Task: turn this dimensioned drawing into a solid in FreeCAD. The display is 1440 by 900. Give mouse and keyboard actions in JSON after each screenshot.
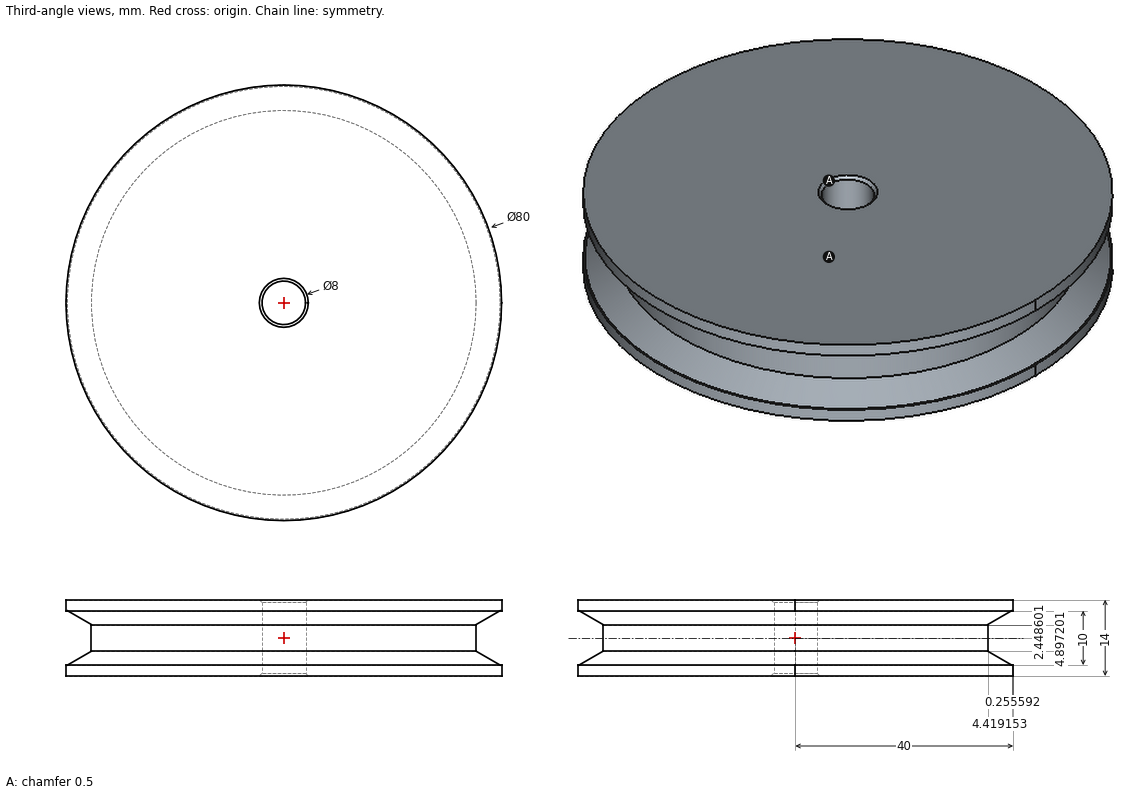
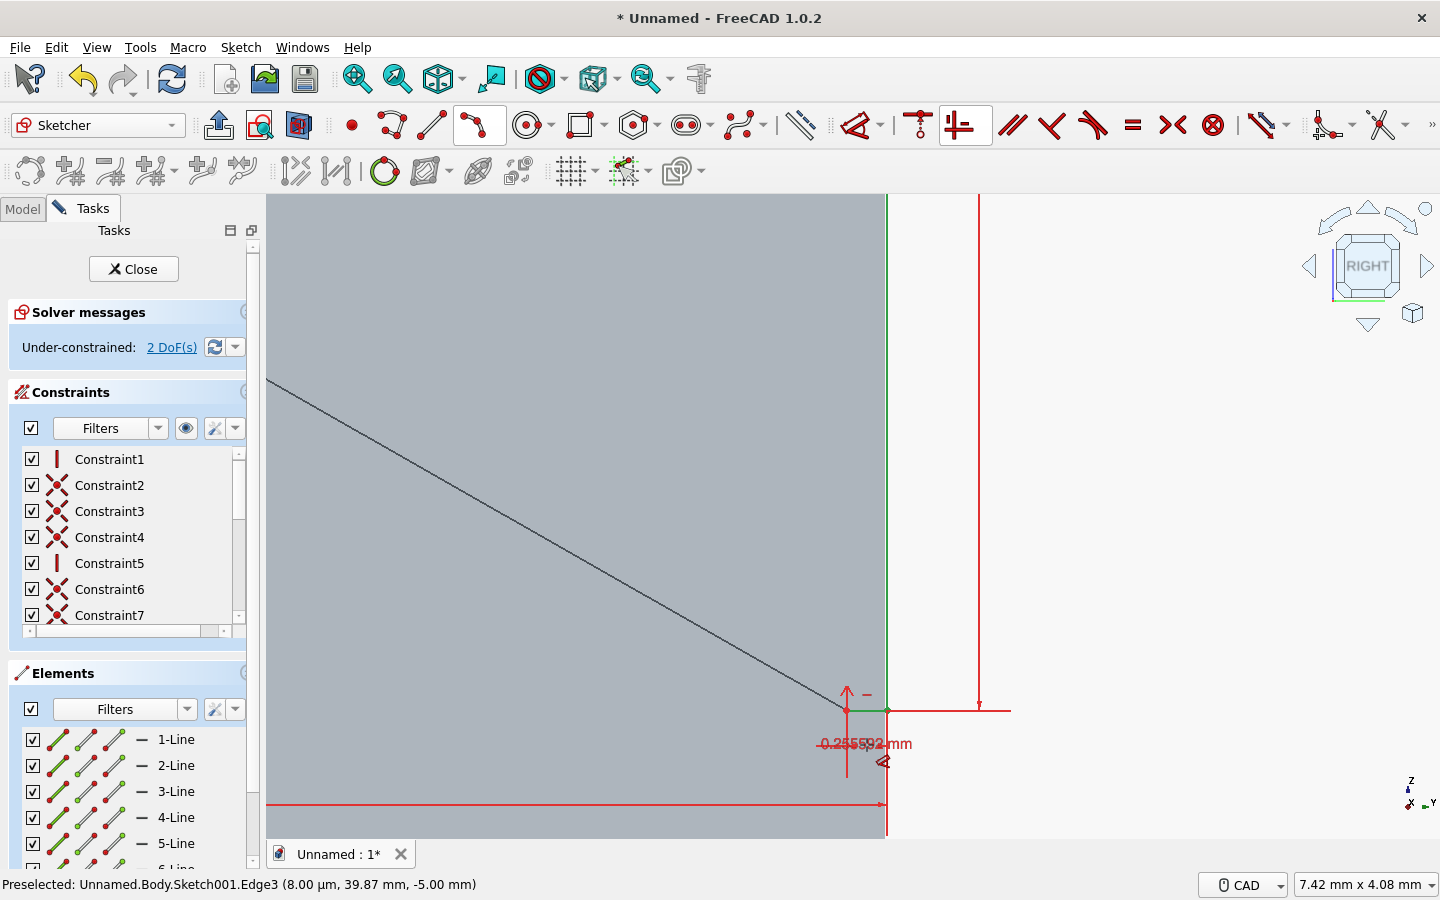
{"action": "scroll", "coordinate": [872, 712], "scroll_direction": "down", "scroll_amount": 7}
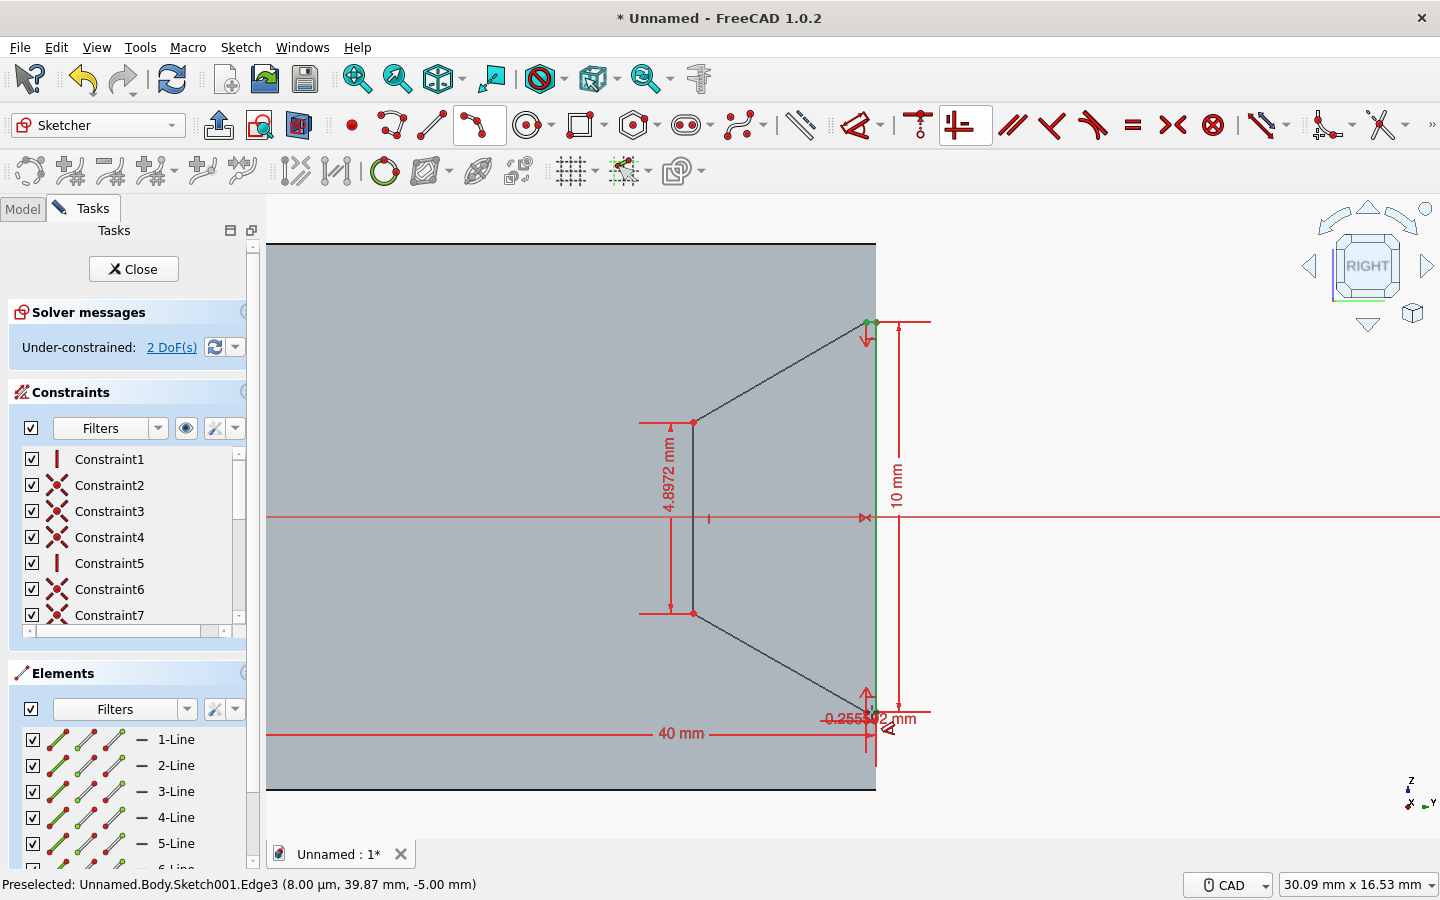
{"action": "left_click", "coordinate": [693, 423]}
{"action": "left_click", "coordinate": [727, 448]}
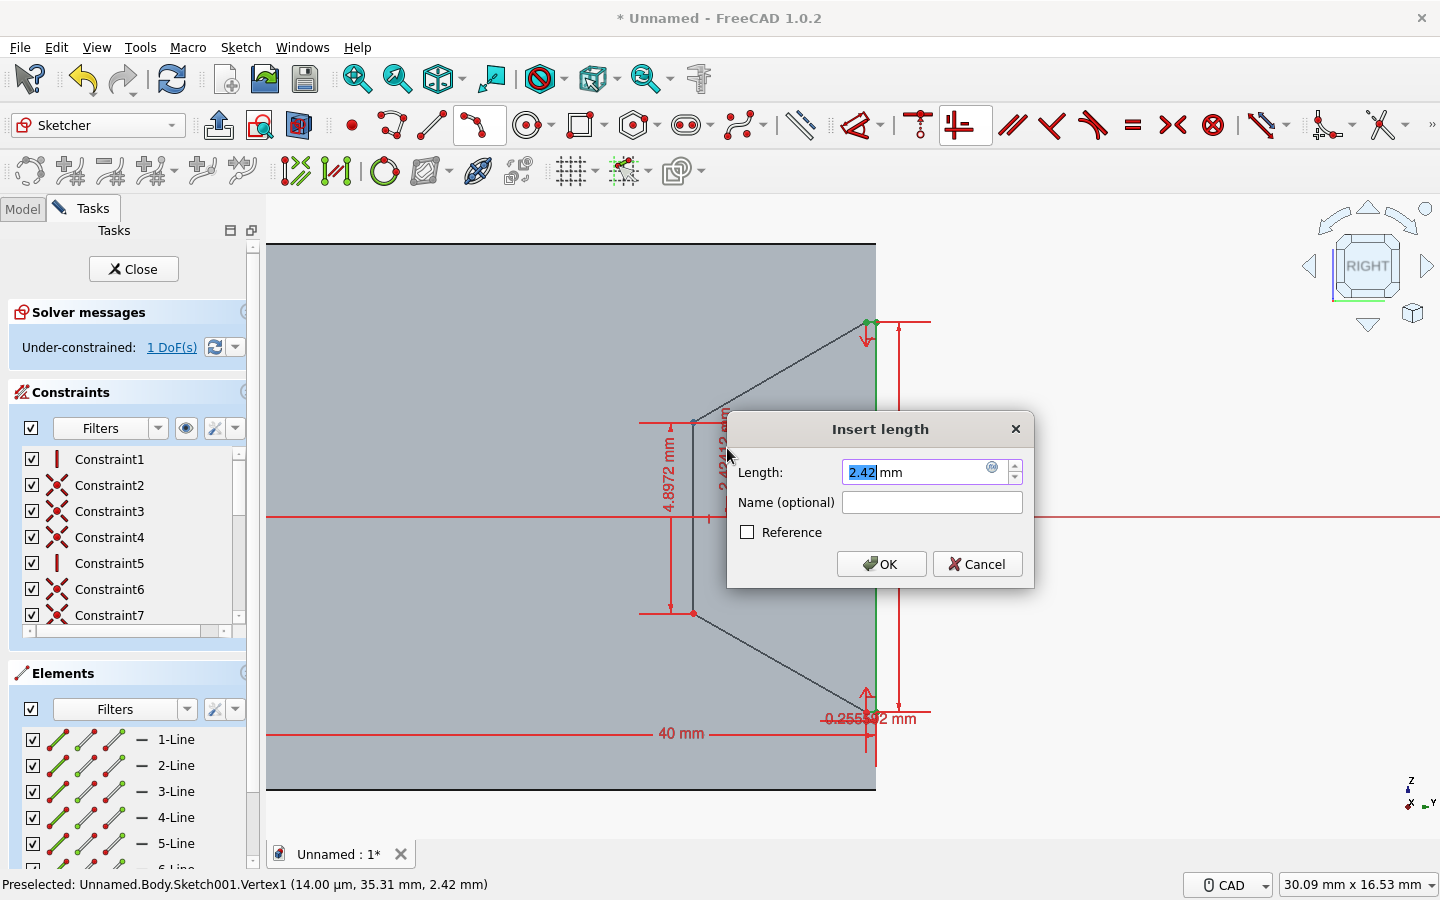
{"action": "type", "text": "2.448601"}
{"action": "key", "text": "Return"}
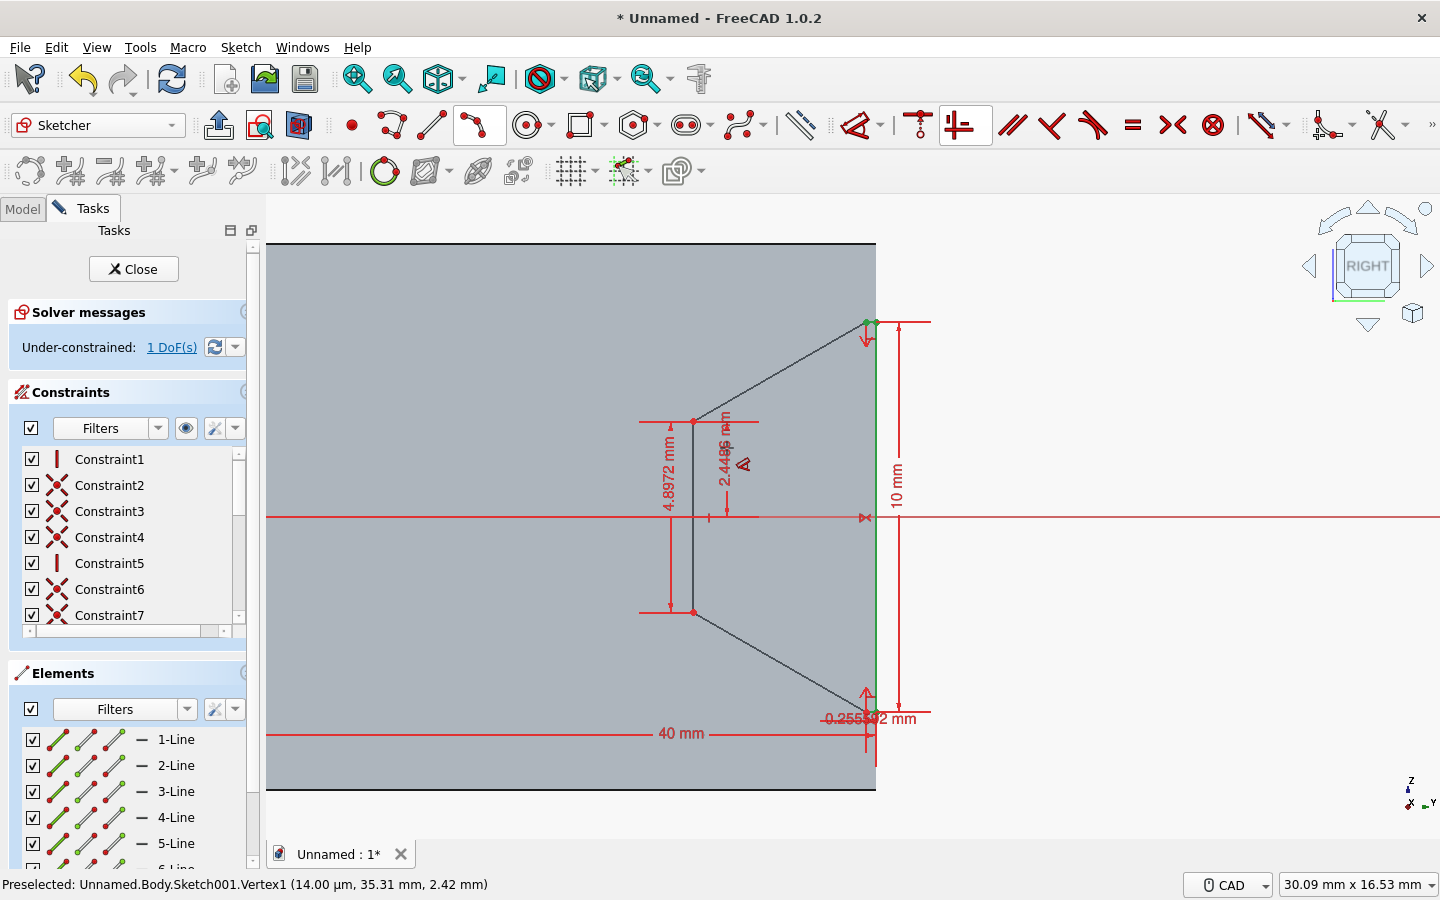
{"action": "left_click", "coordinate": [745, 643]}
{"action": "left_click", "coordinate": [780, 746]}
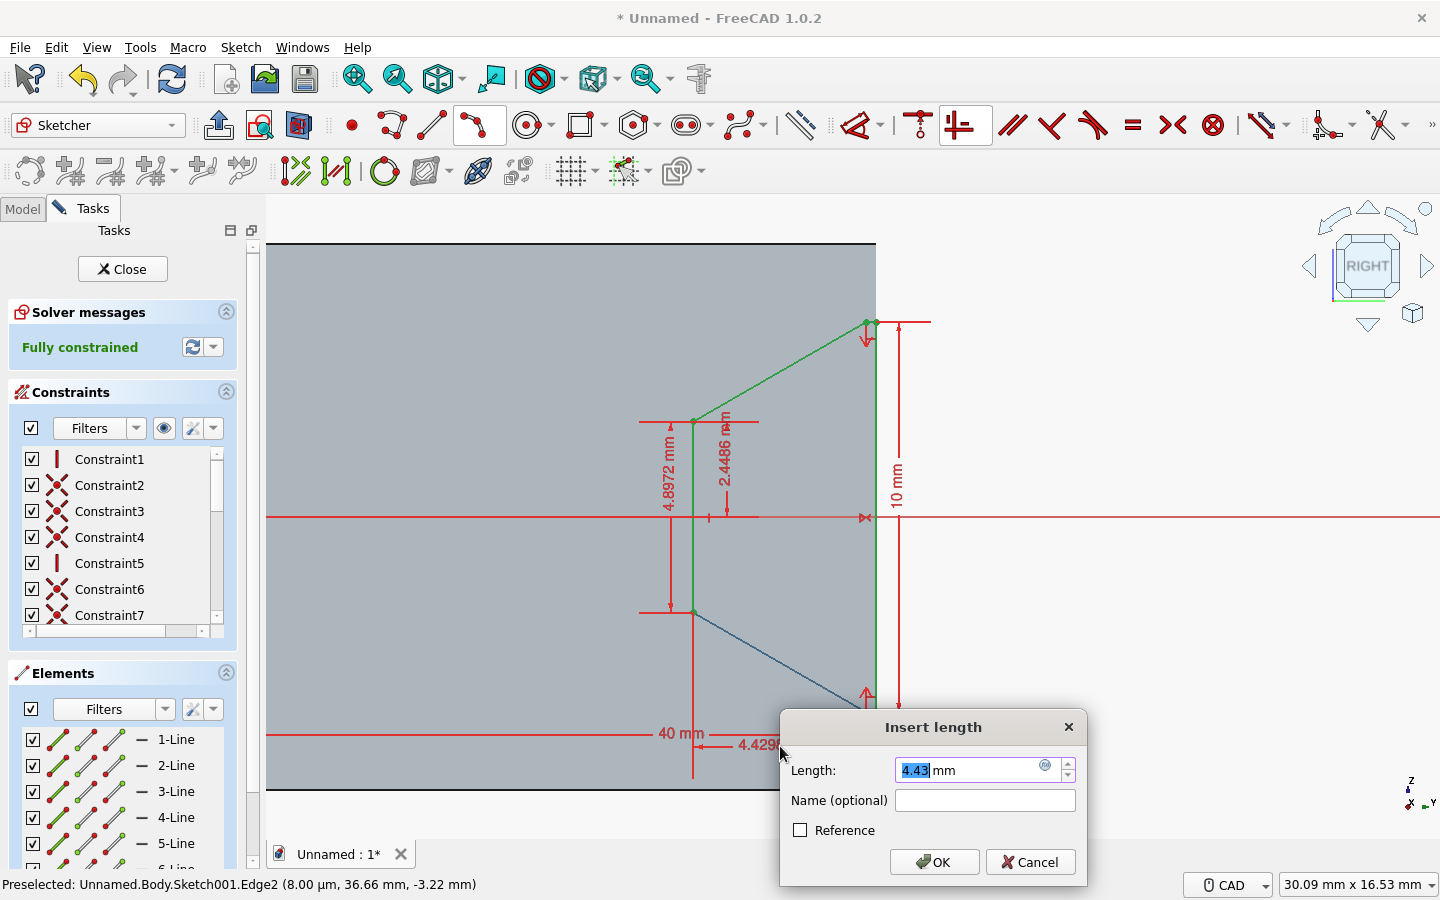
{"action": "type", "text": "4.419153"}
{"action": "key", "text": "Return"}
{"action": "key", "text": "Escape"}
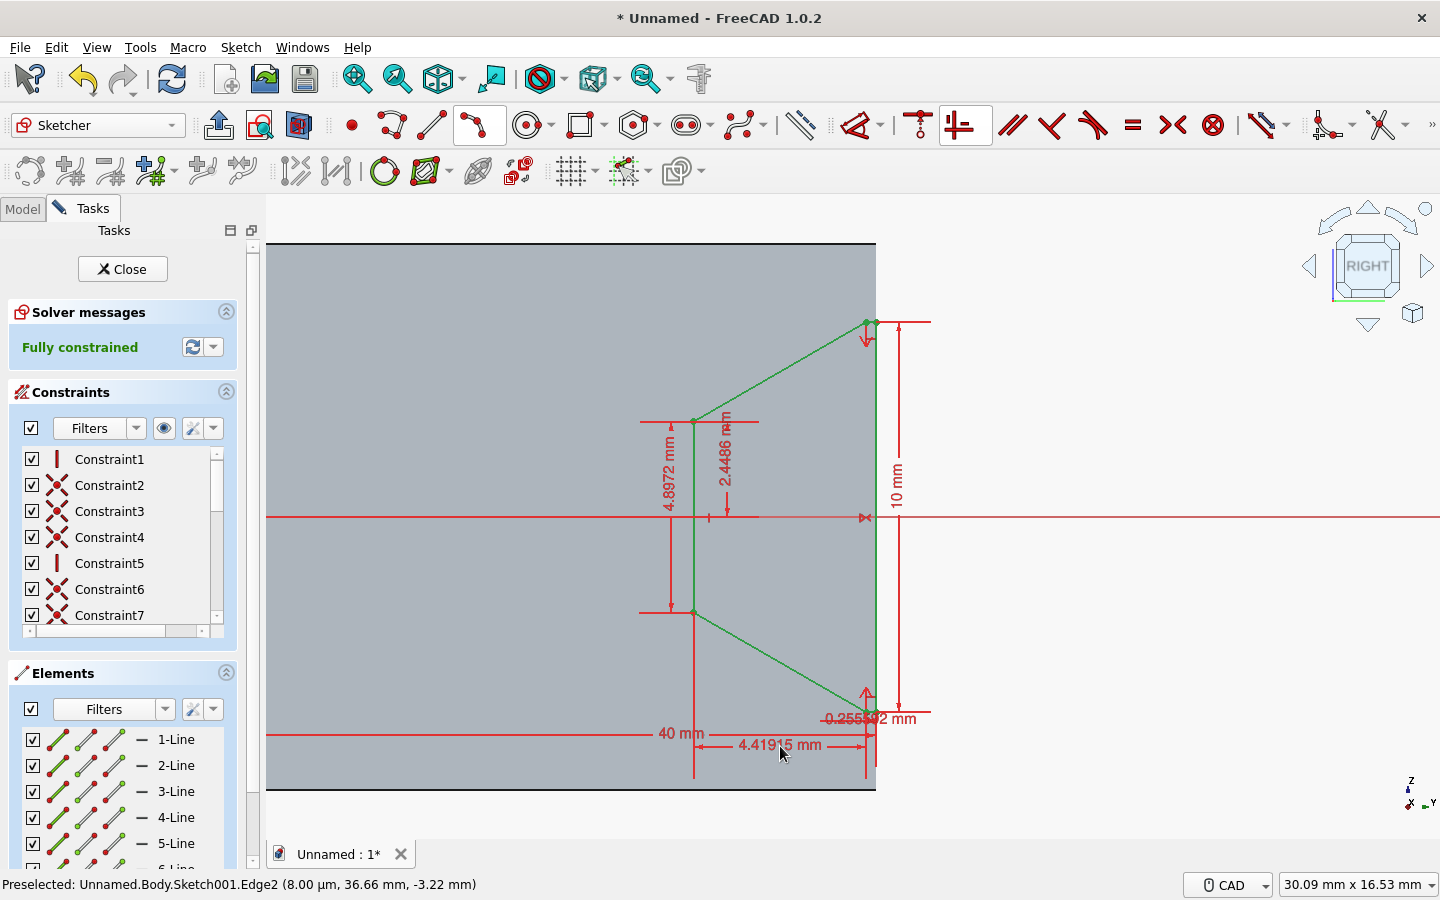
{"action": "left_click", "coordinate": [123, 269]}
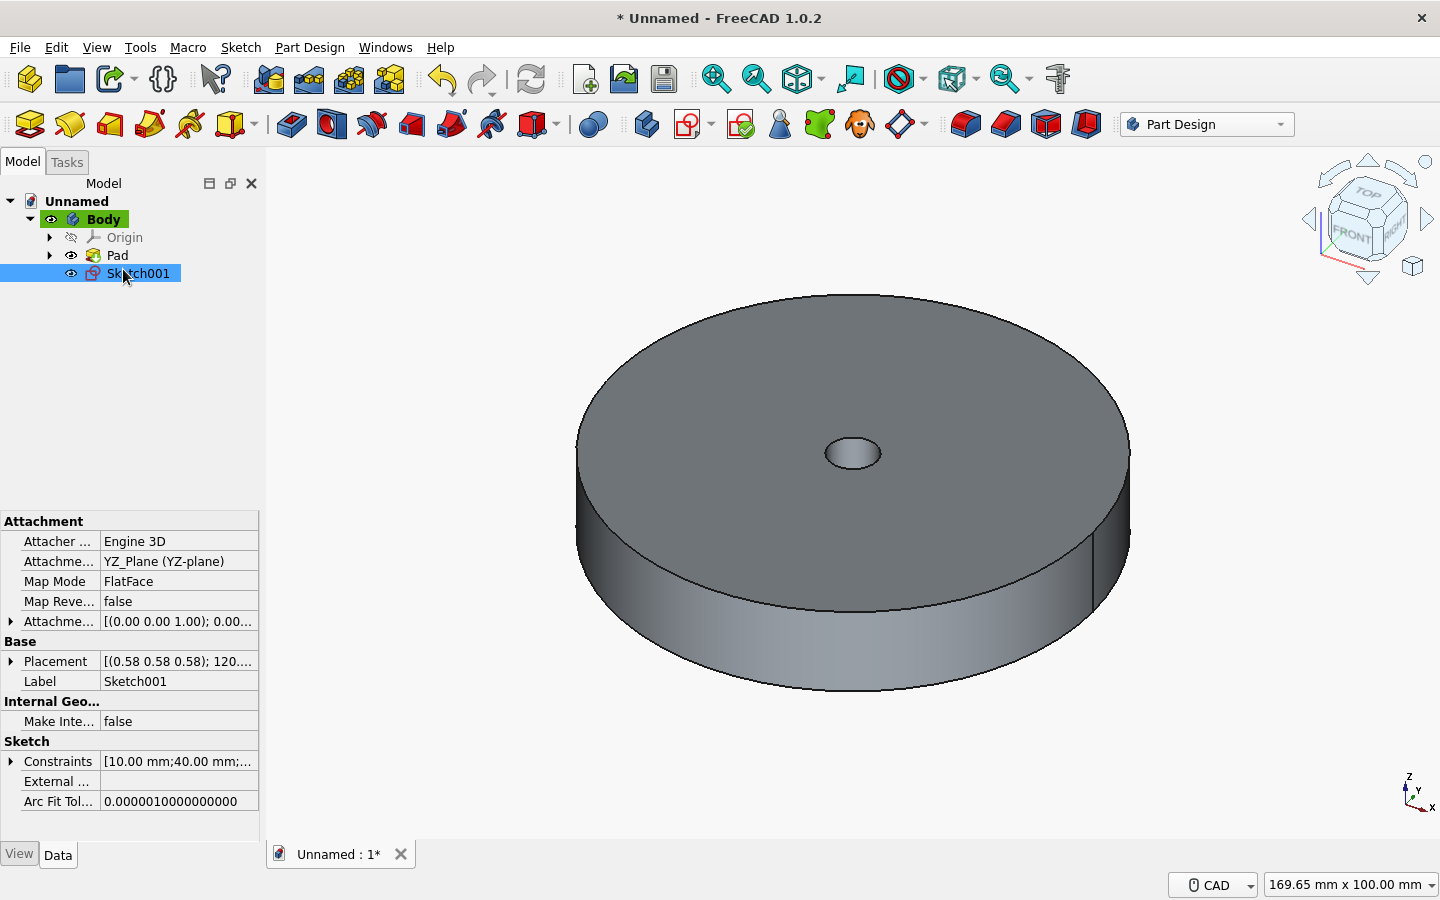
{"action": "left_click", "coordinate": [372, 124]}